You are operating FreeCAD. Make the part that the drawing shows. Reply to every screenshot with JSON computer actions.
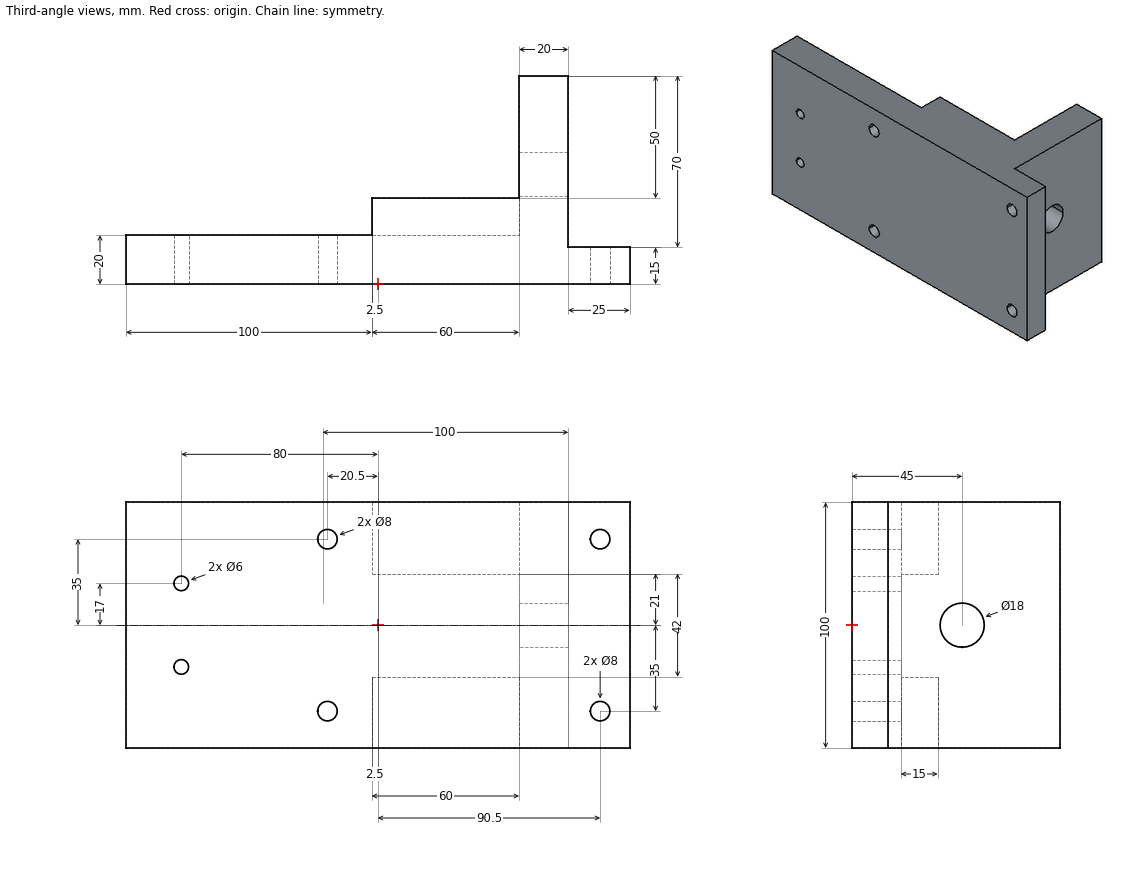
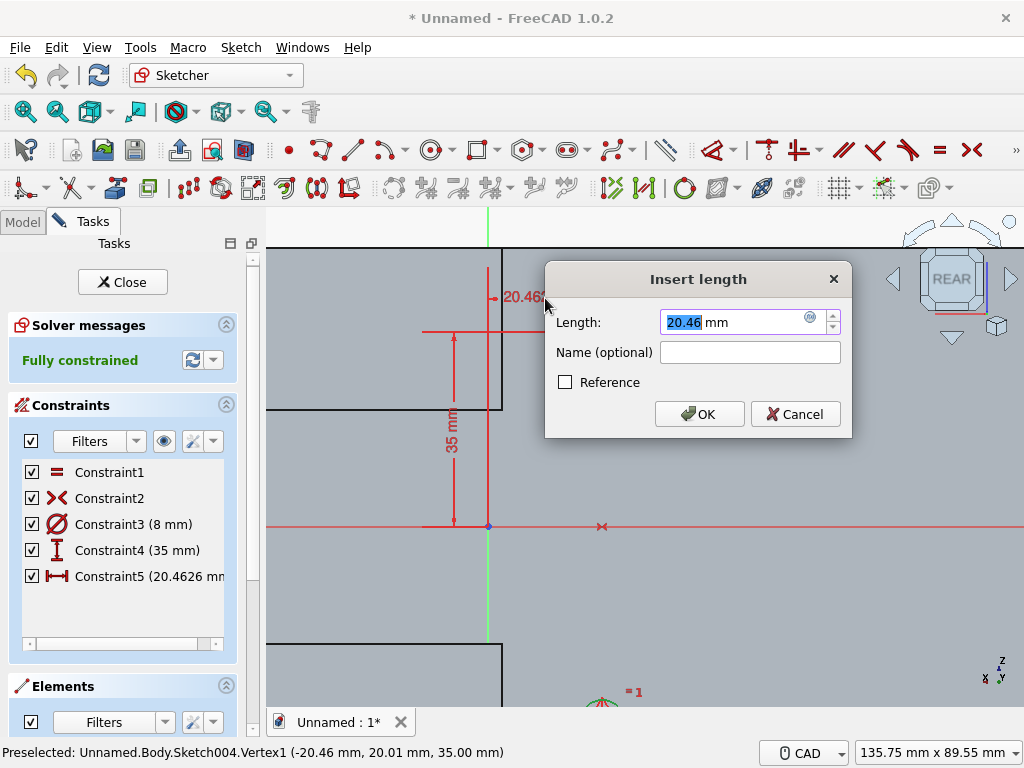
{"action": "type", "text": "20.5"}
{"action": "key", "text": "Return"}
{"action": "key", "text": "Escape"}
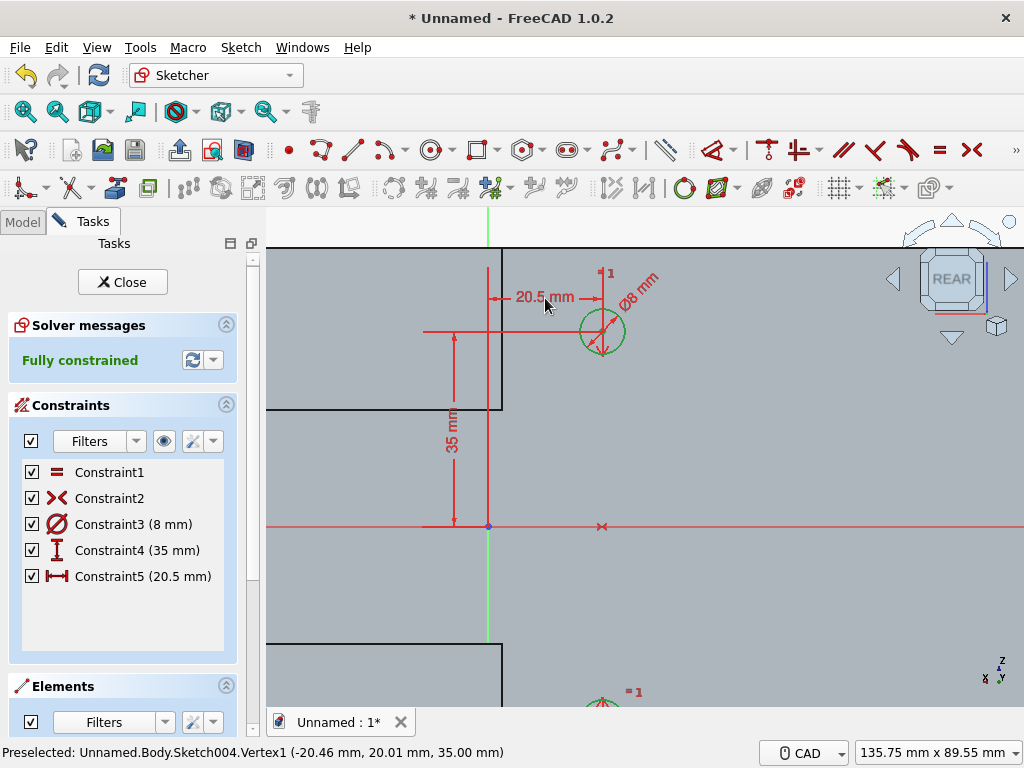
{"action": "left_click", "coordinate": [123, 282]}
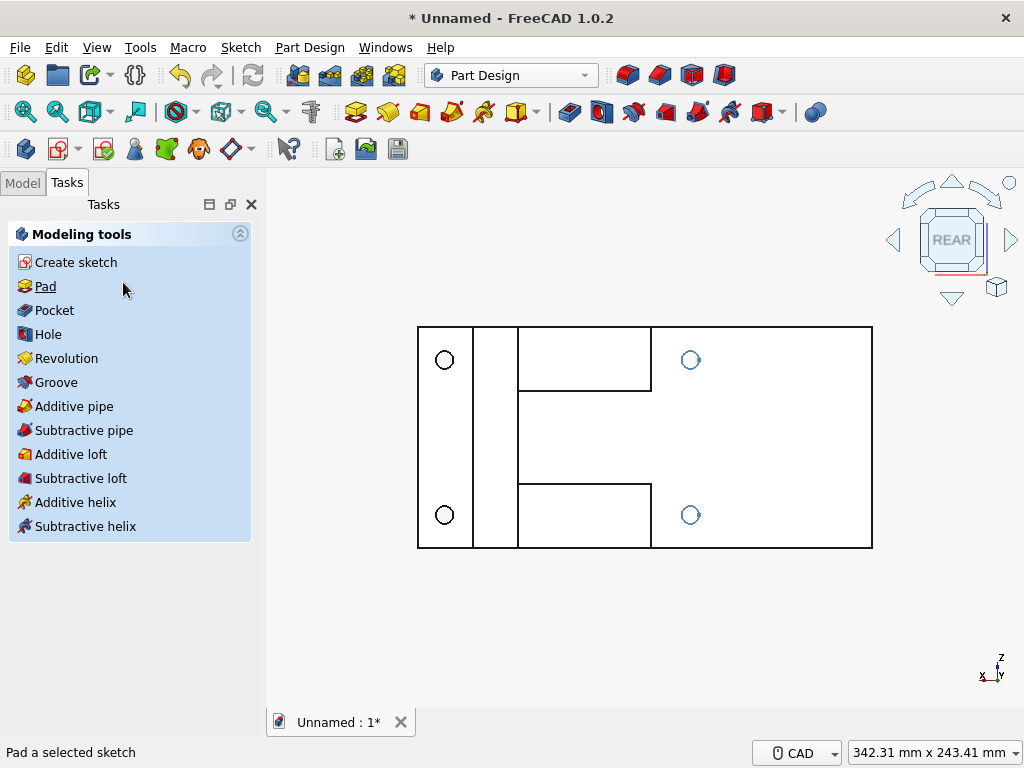
{"action": "left_click", "coordinate": [570, 112]}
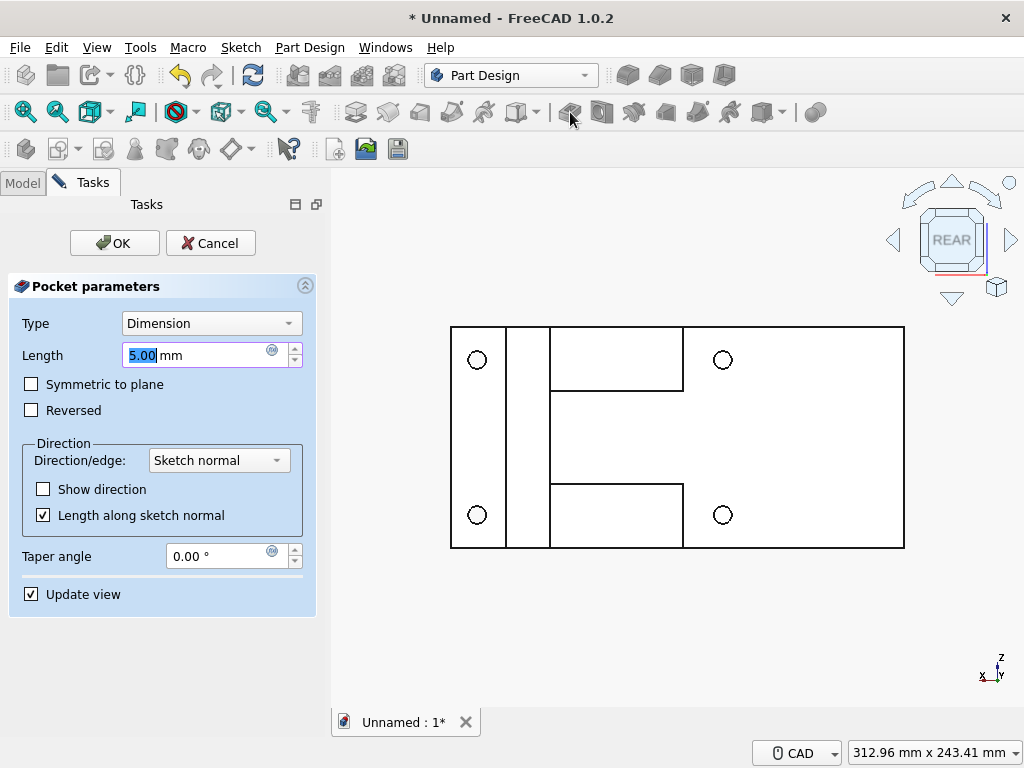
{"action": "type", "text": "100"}
{"action": "key", "text": "Tab"}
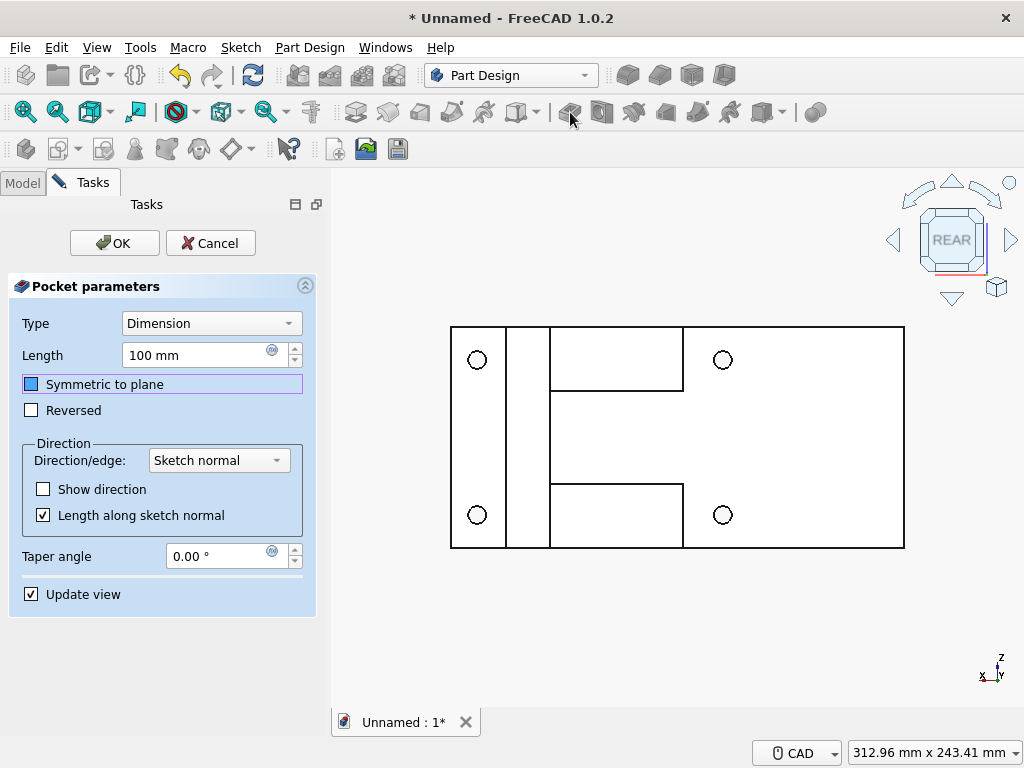
{"action": "left_click", "coordinate": [115, 243]}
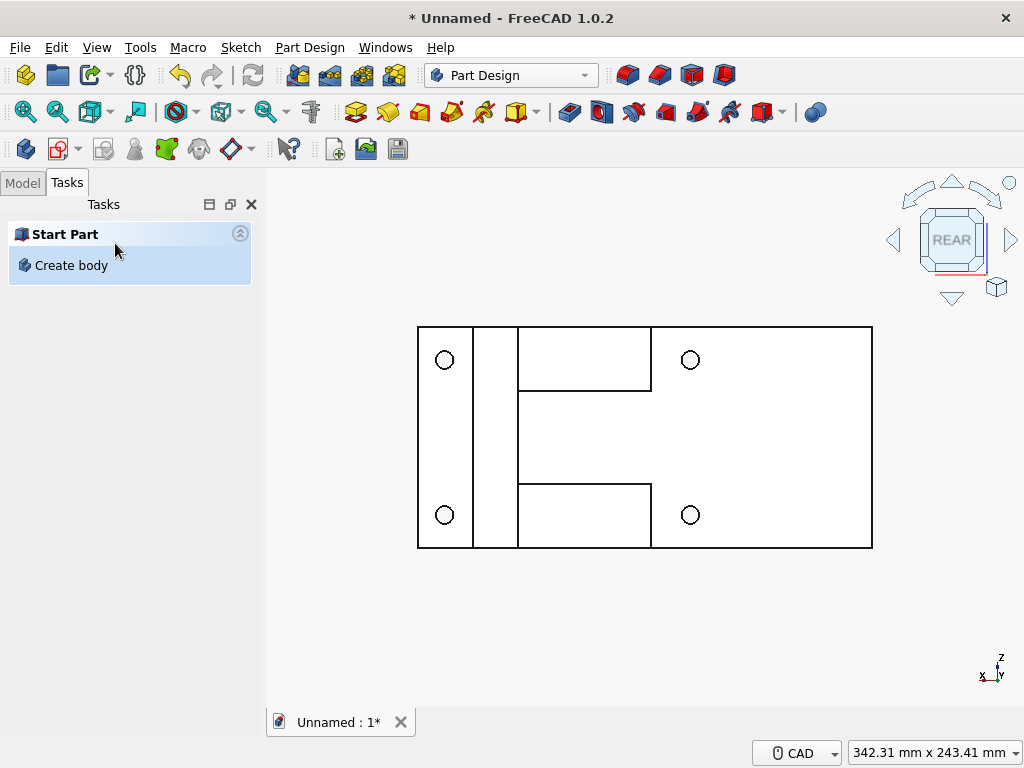
{"action": "left_click", "coordinate": [745, 437]}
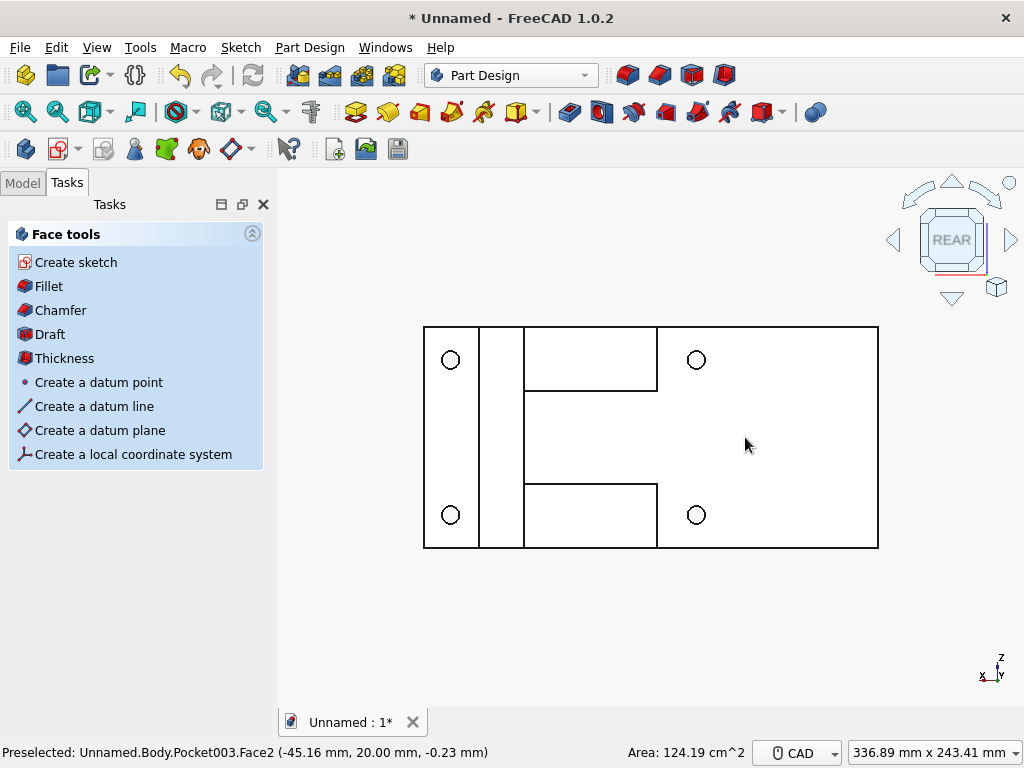
{"action": "left_click", "coordinate": [58, 150]}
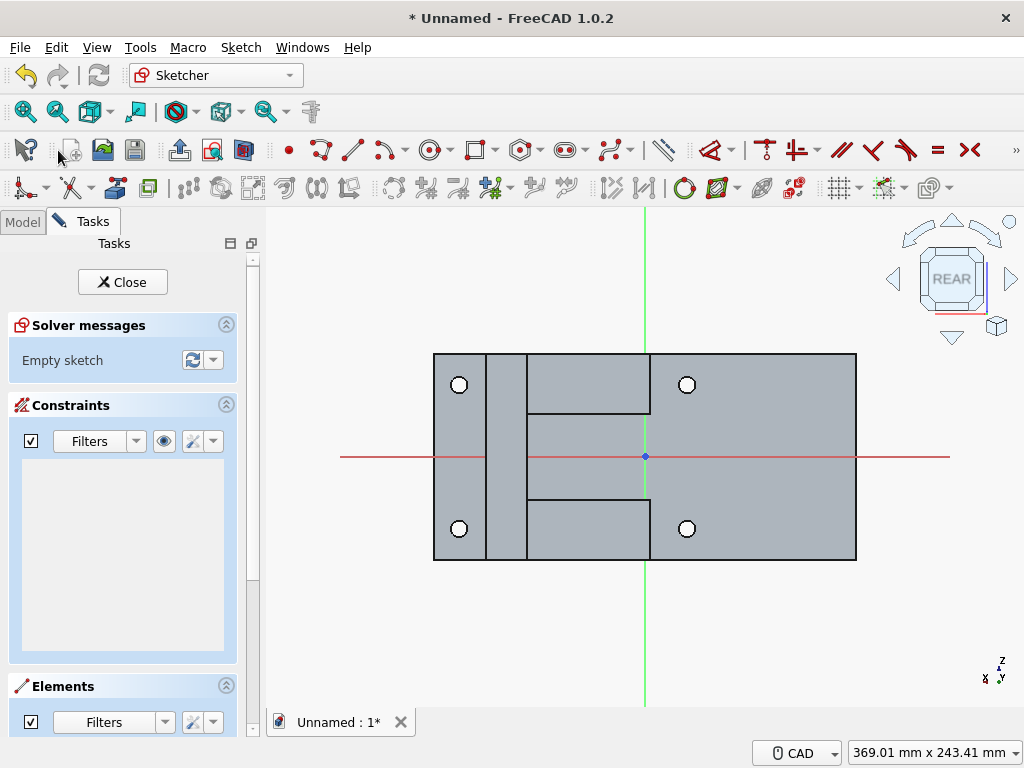
{"action": "scroll", "coordinate": [856, 457], "scroll_direction": "up", "scroll_amount": 4}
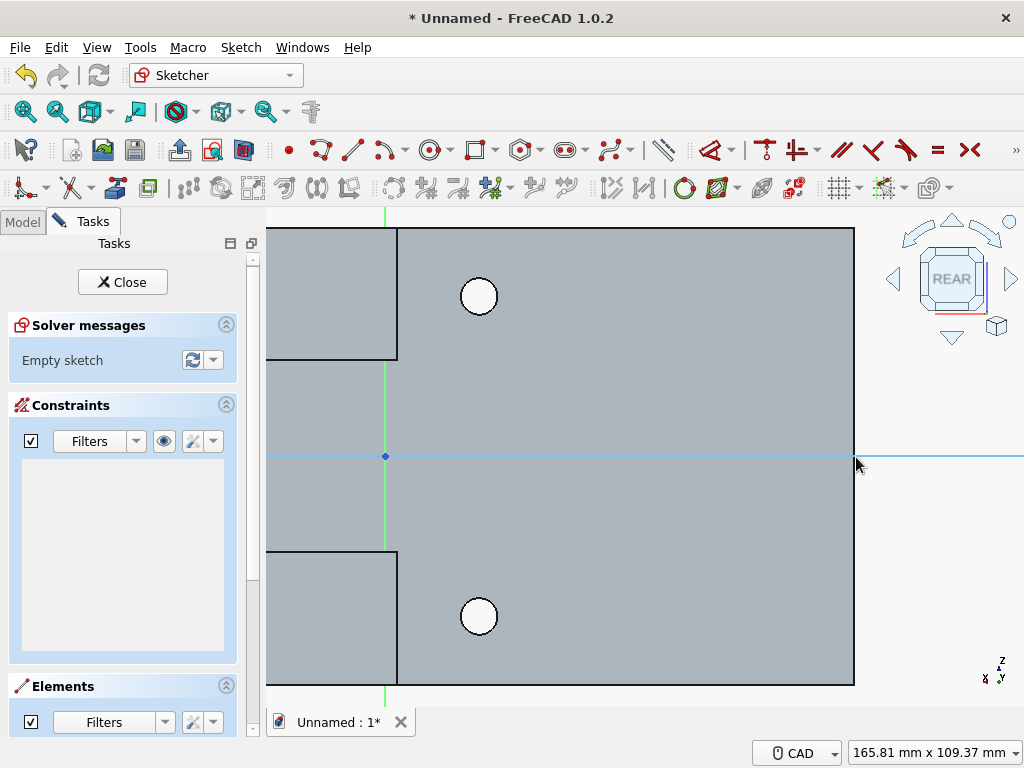
{"action": "left_click", "coordinate": [430, 150]}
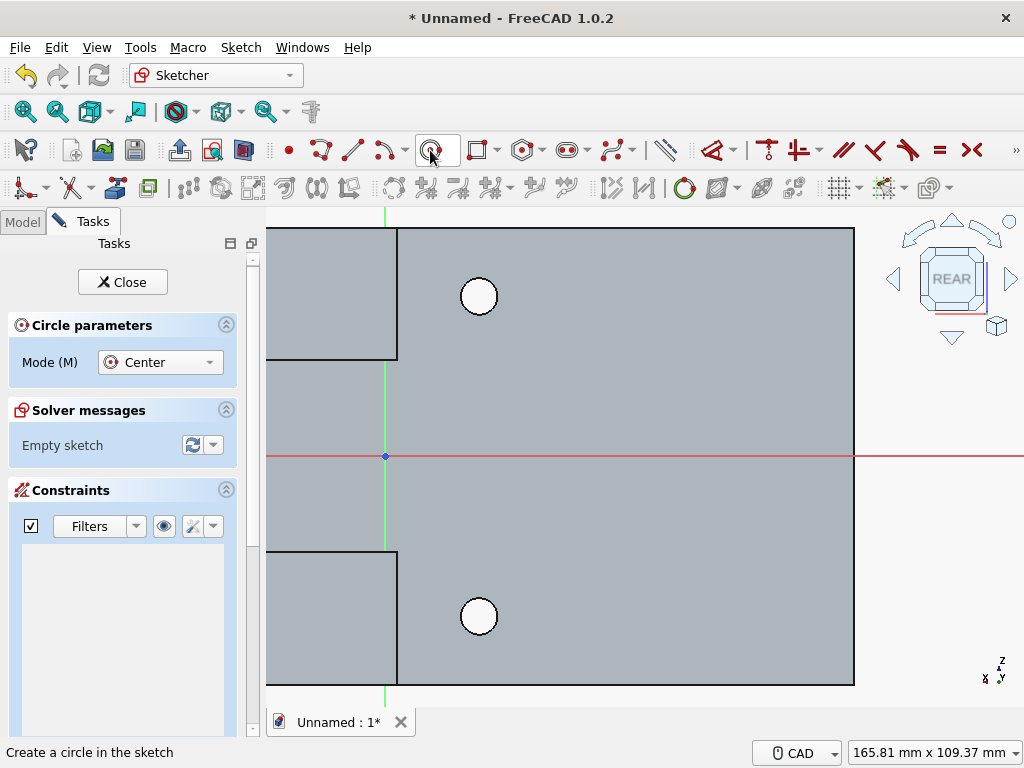
{"action": "scroll", "coordinate": [751, 379], "scroll_direction": "up", "scroll_amount": 3}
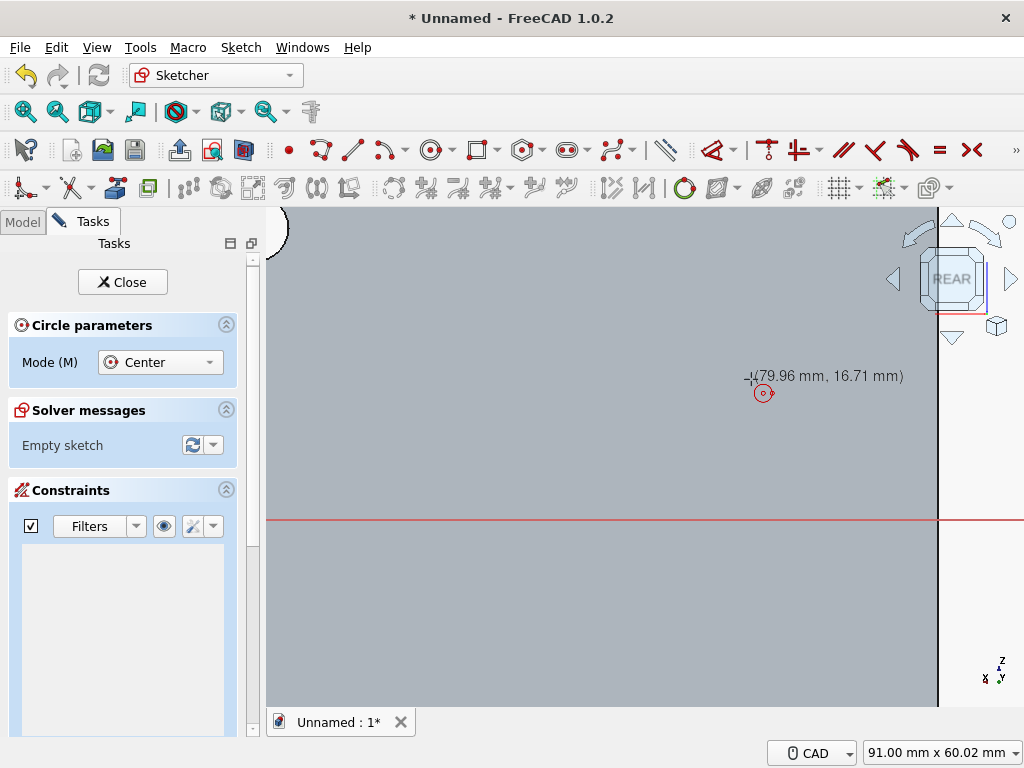
{"action": "left_click", "coordinate": [751, 378]}
{"action": "left_click", "coordinate": [768, 360]}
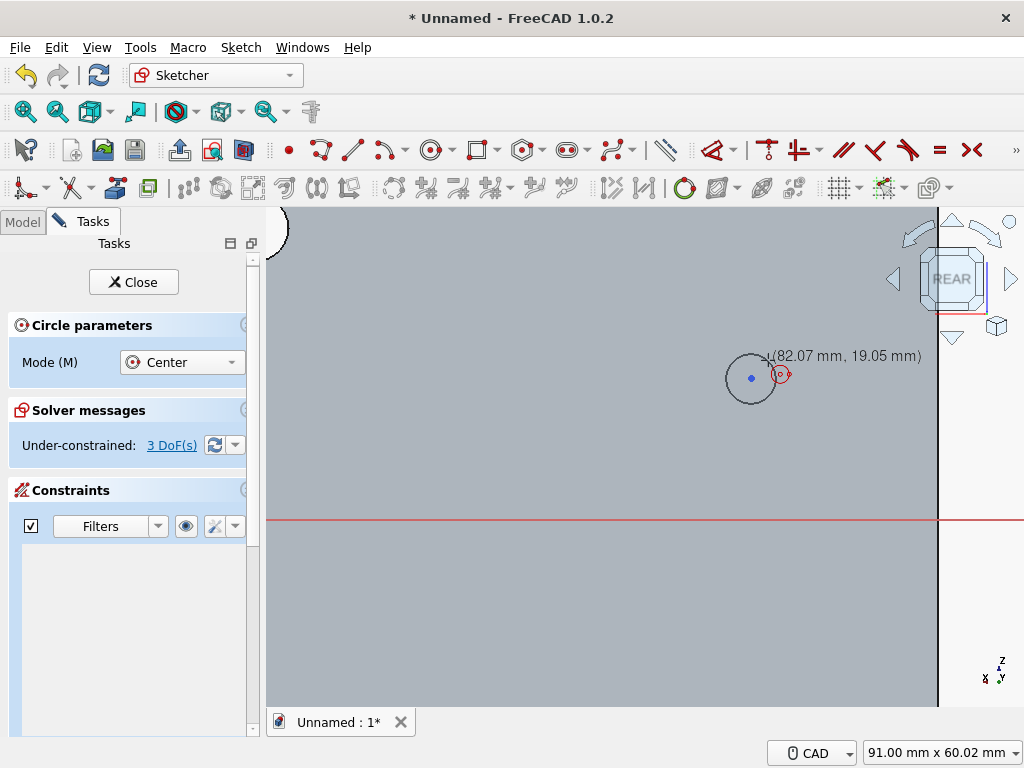
{"action": "left_click", "coordinate": [751, 661]}
{"action": "left_click", "coordinate": [768, 644]}
{"action": "key", "text": "Escape"}